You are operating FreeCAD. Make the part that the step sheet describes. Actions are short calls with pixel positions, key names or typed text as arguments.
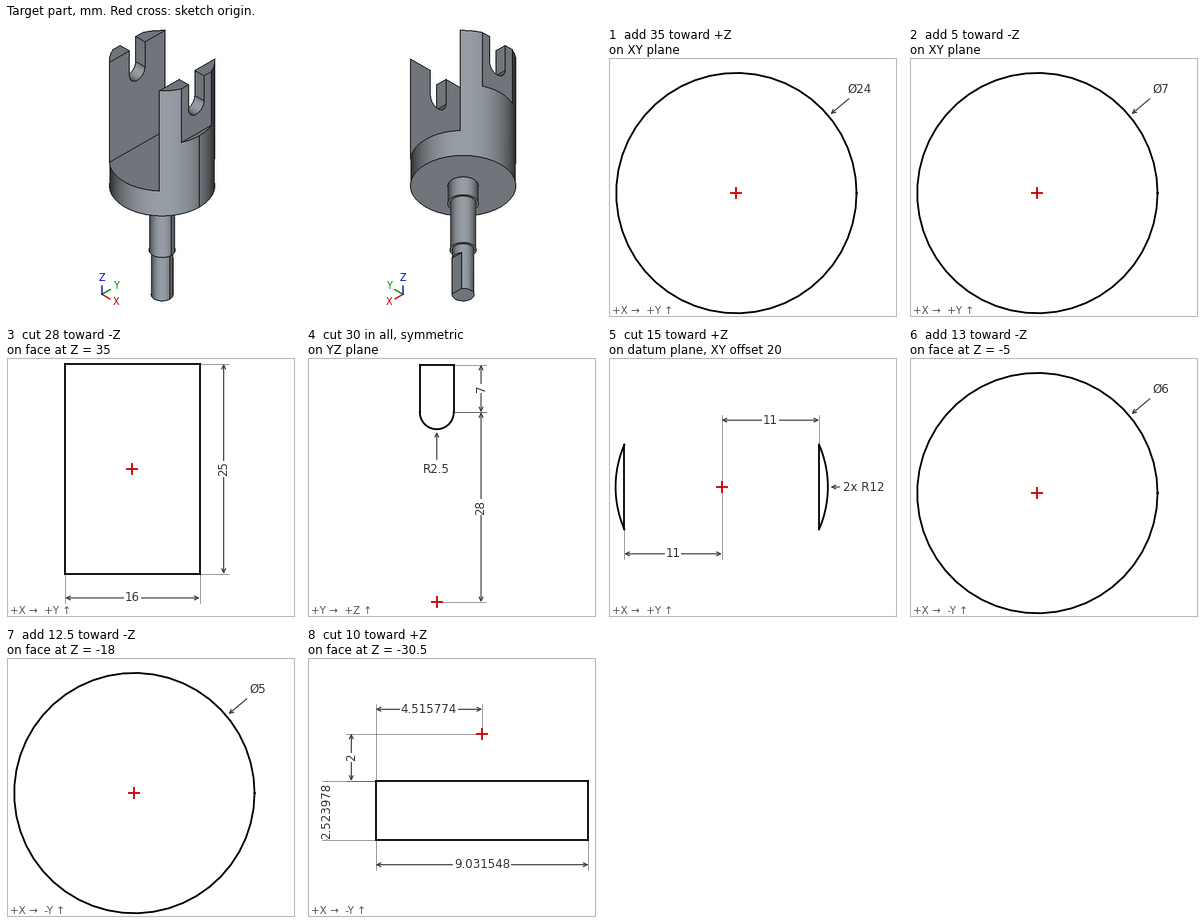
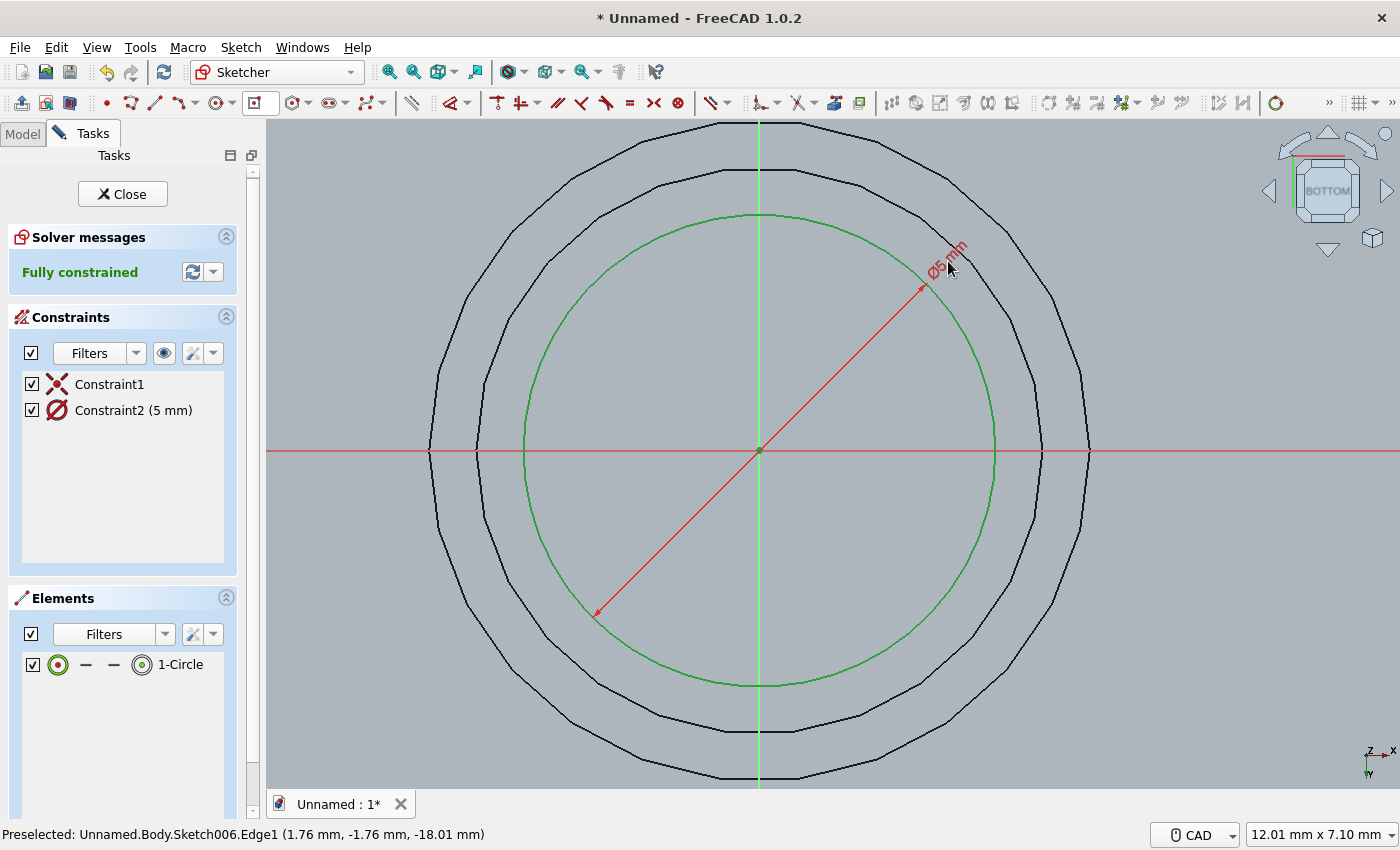
click(123, 194)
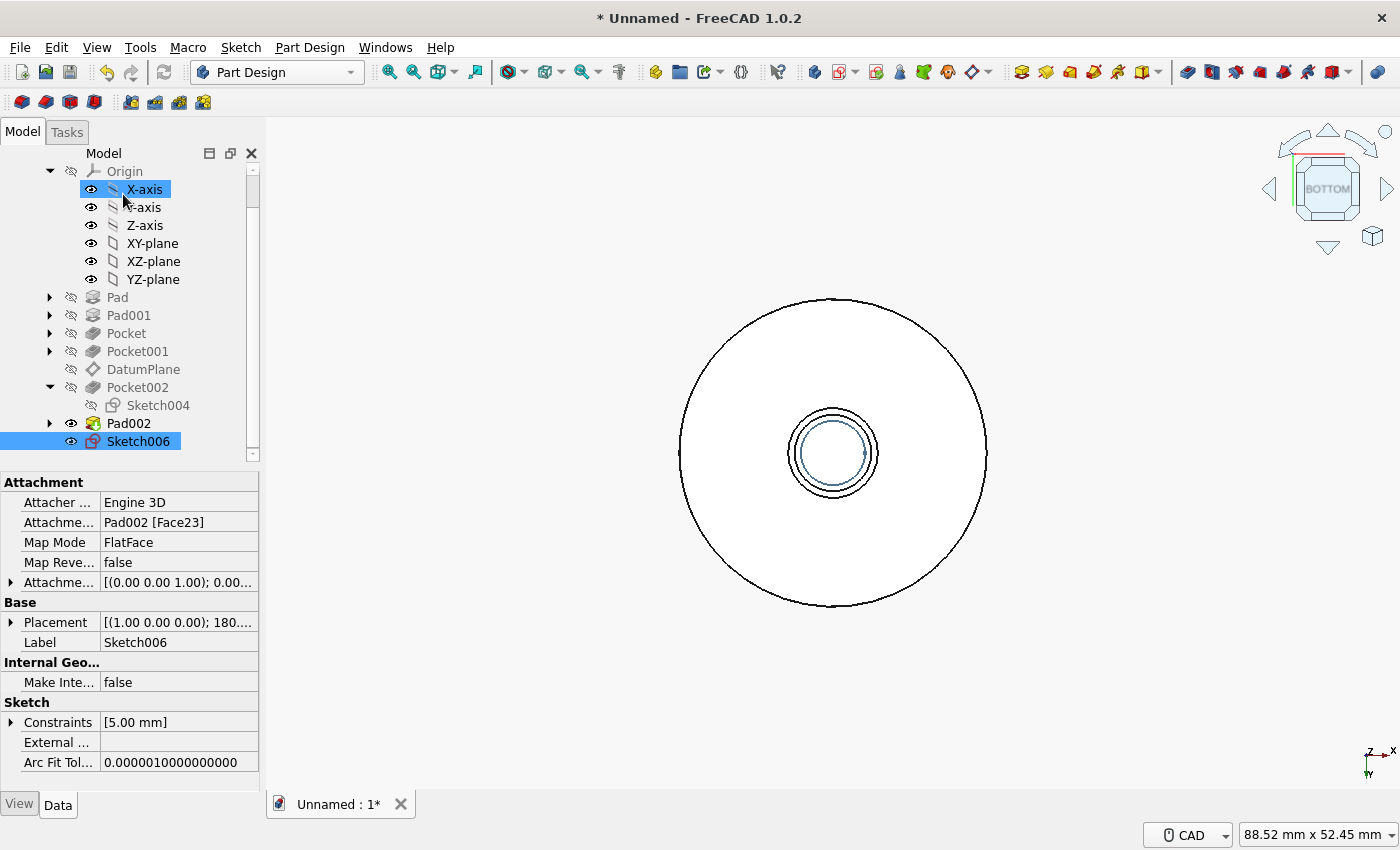
click(1022, 72)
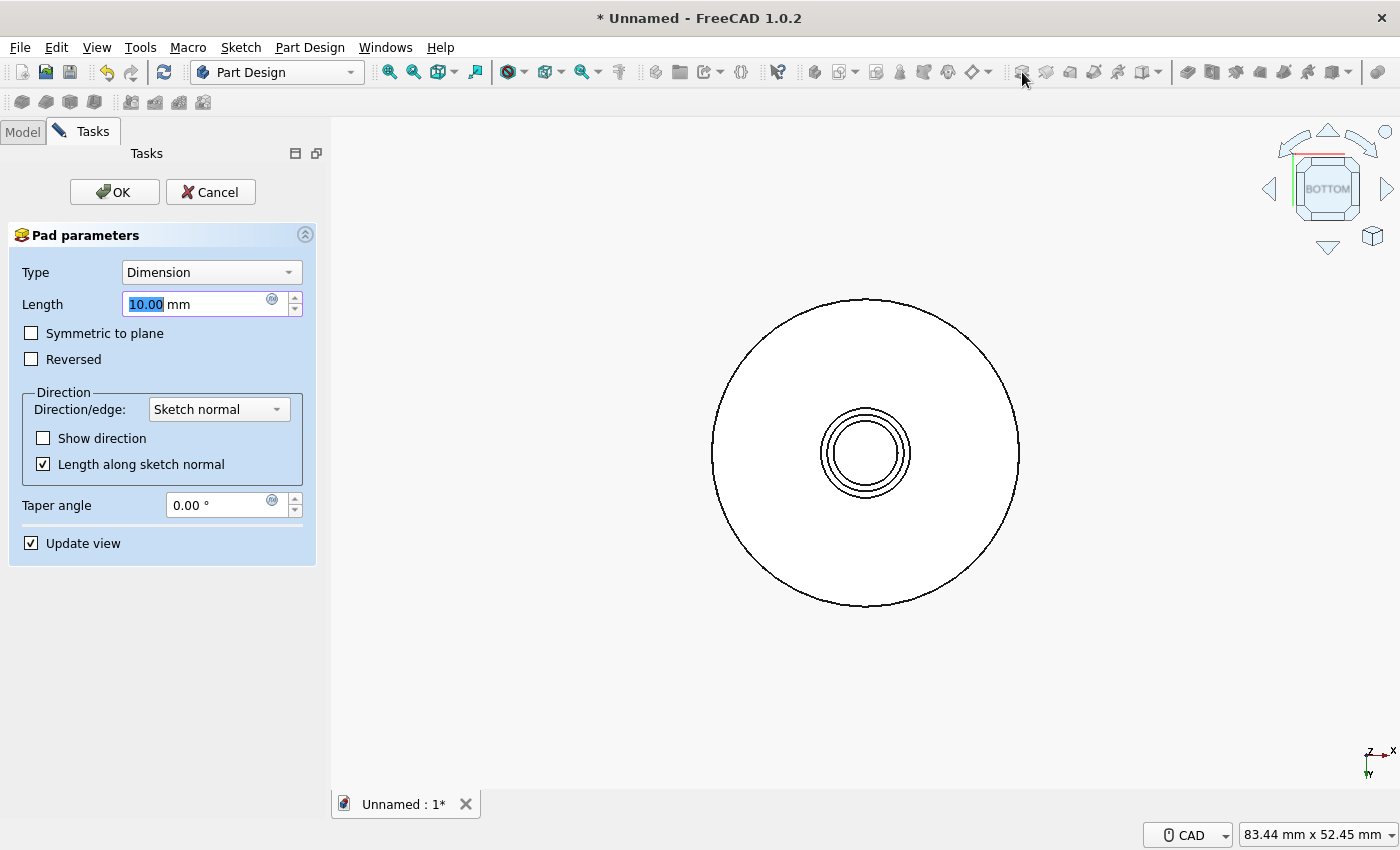
text(12.5)
key(Tab)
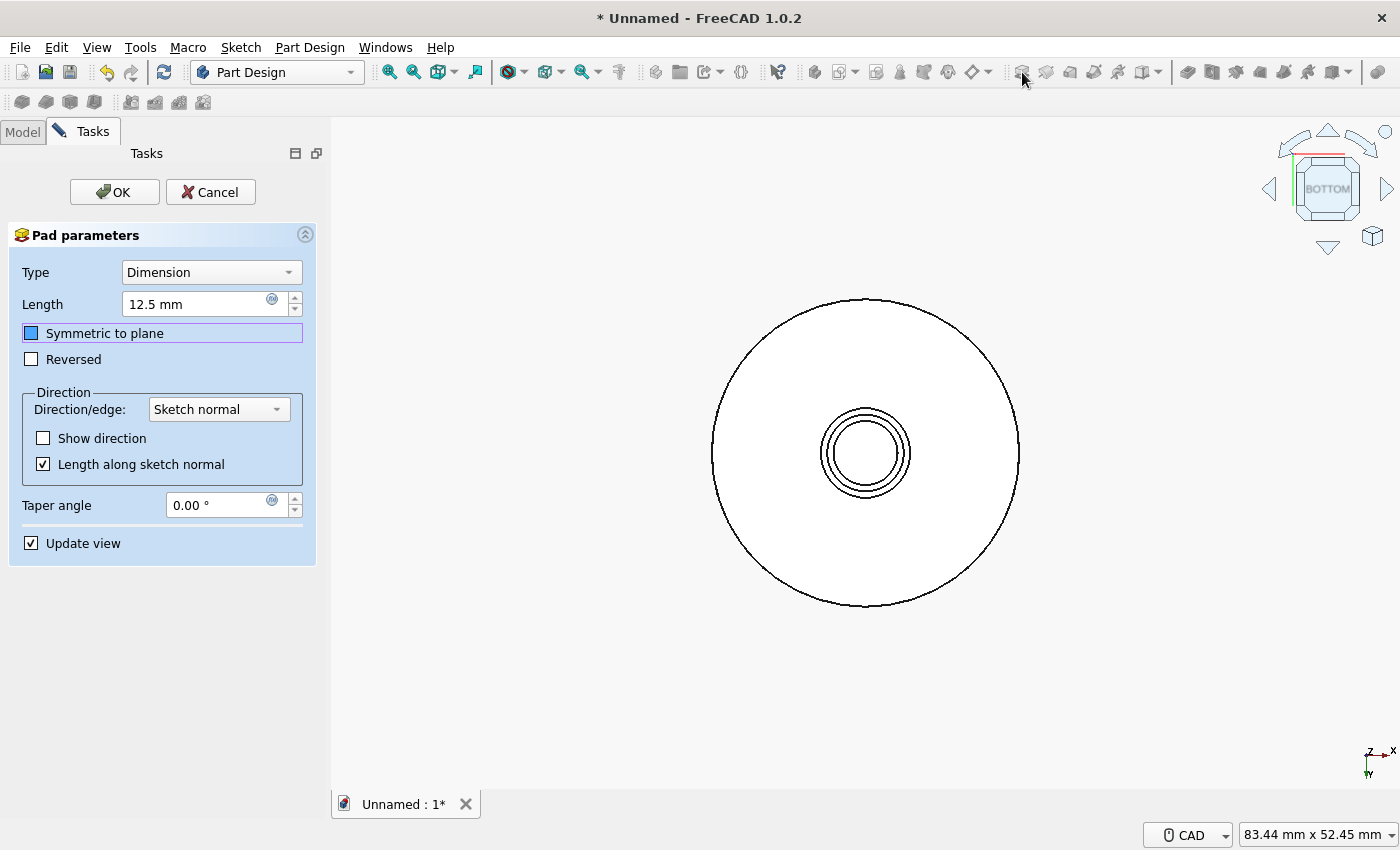
click(115, 192)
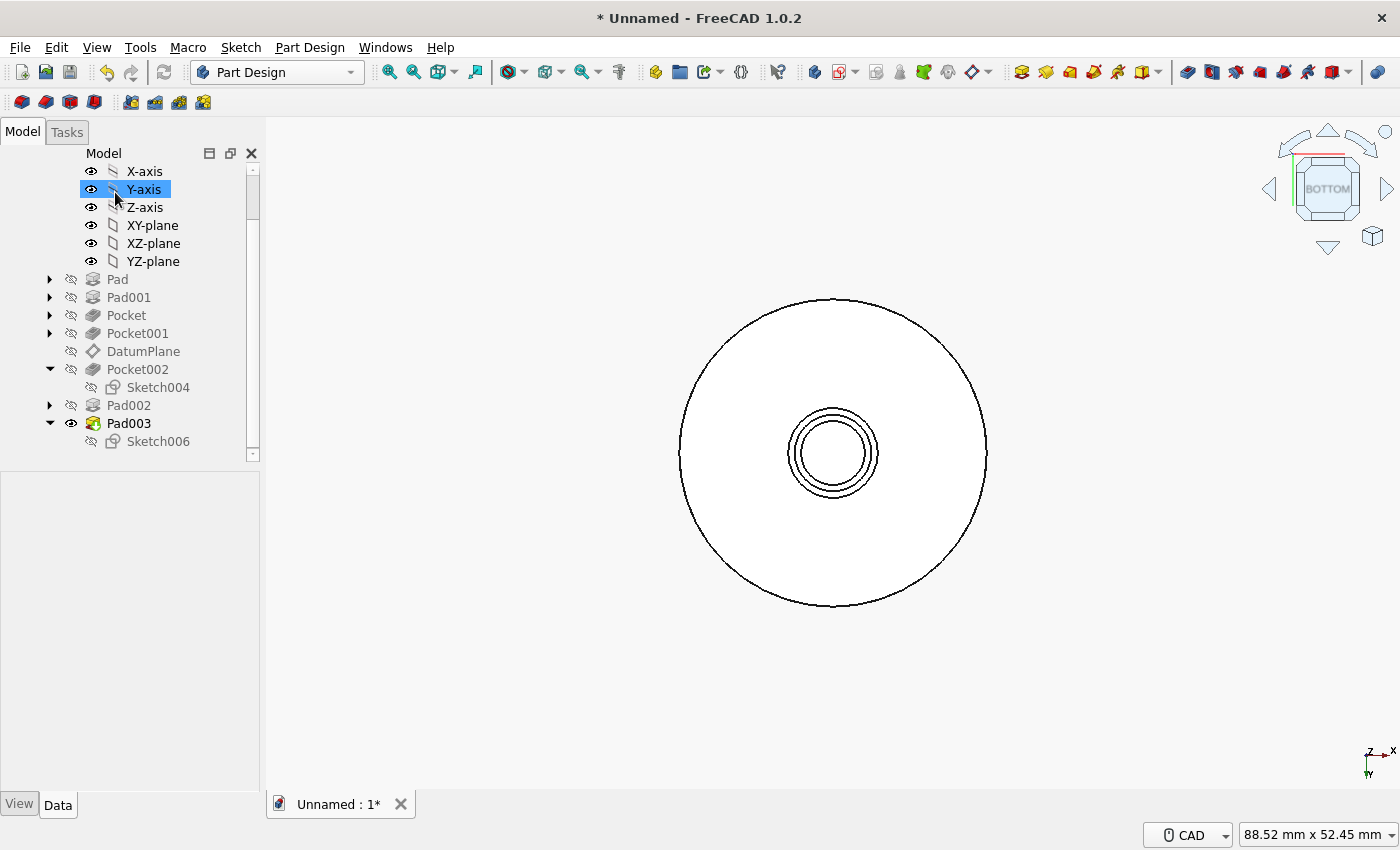
click(833, 452)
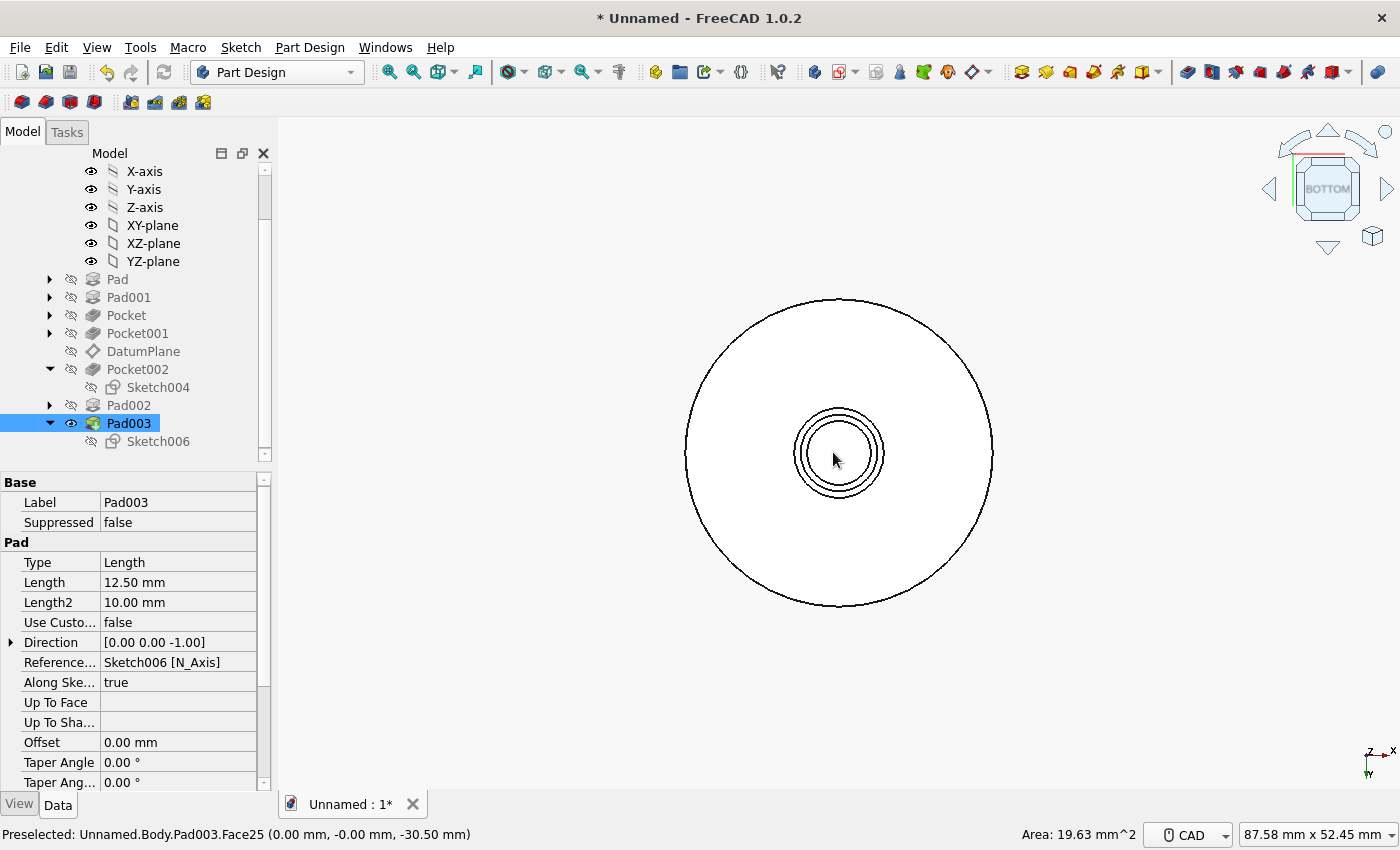
click(840, 72)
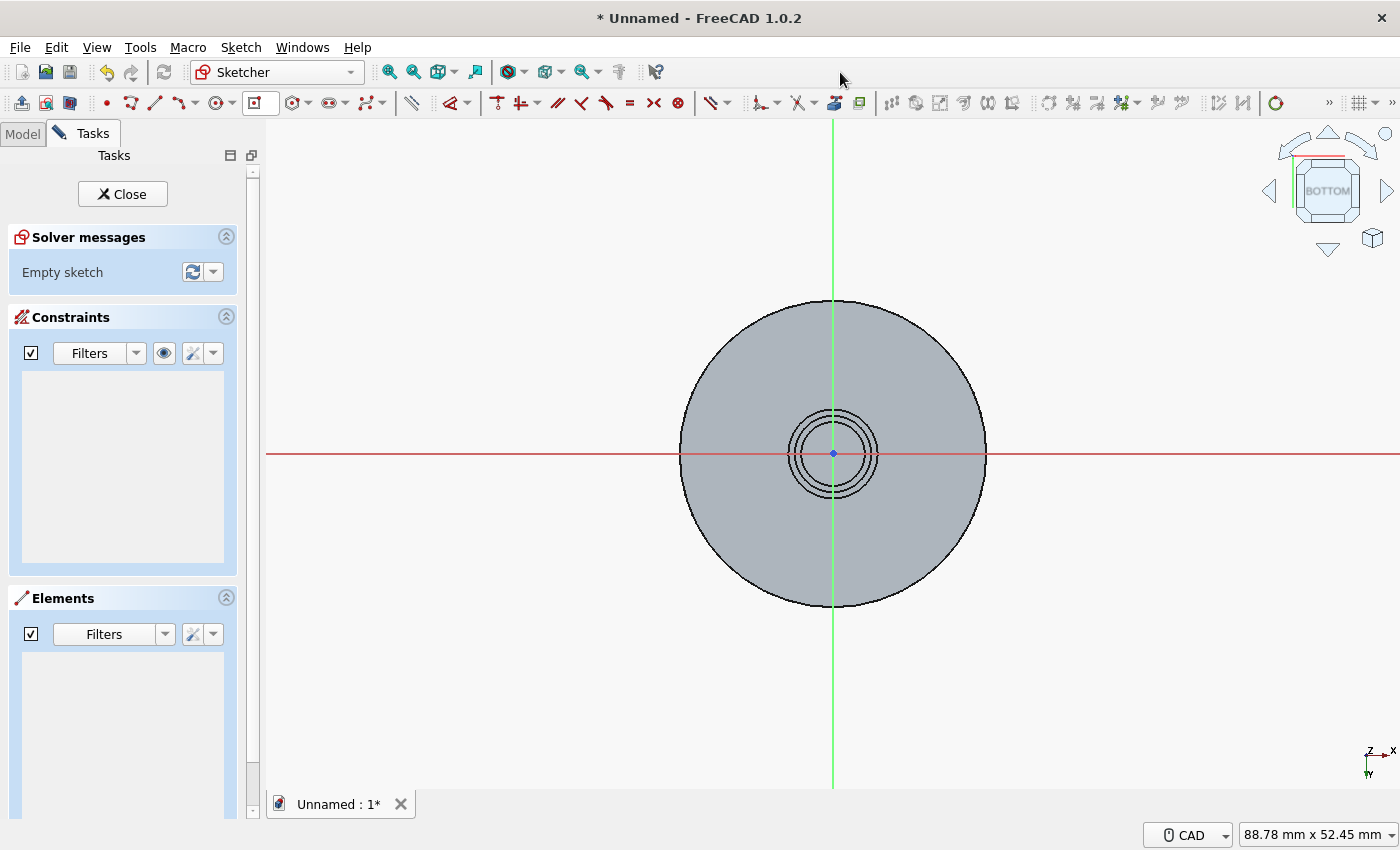
scroll(847, 489, up, 9)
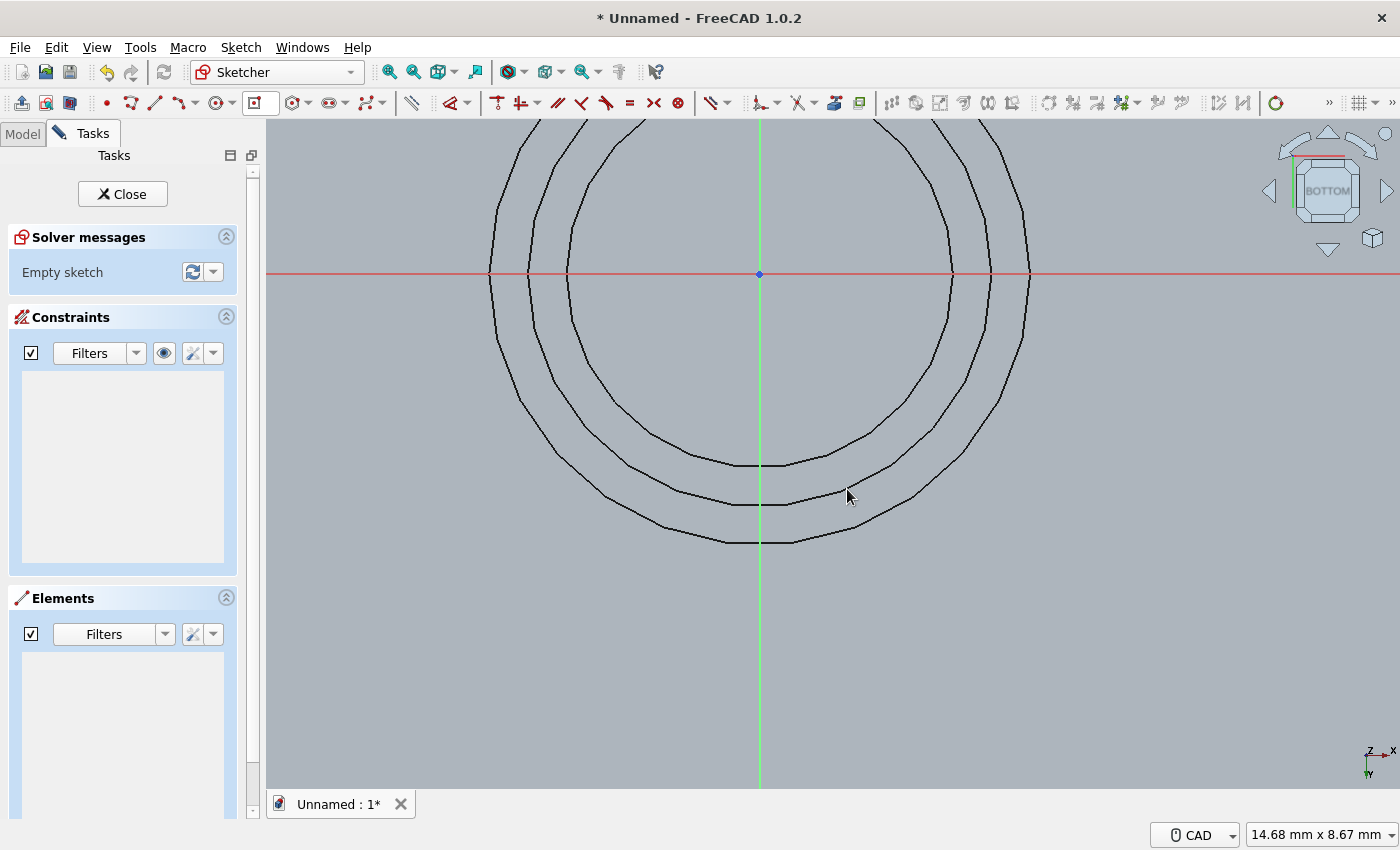
click(274, 104)